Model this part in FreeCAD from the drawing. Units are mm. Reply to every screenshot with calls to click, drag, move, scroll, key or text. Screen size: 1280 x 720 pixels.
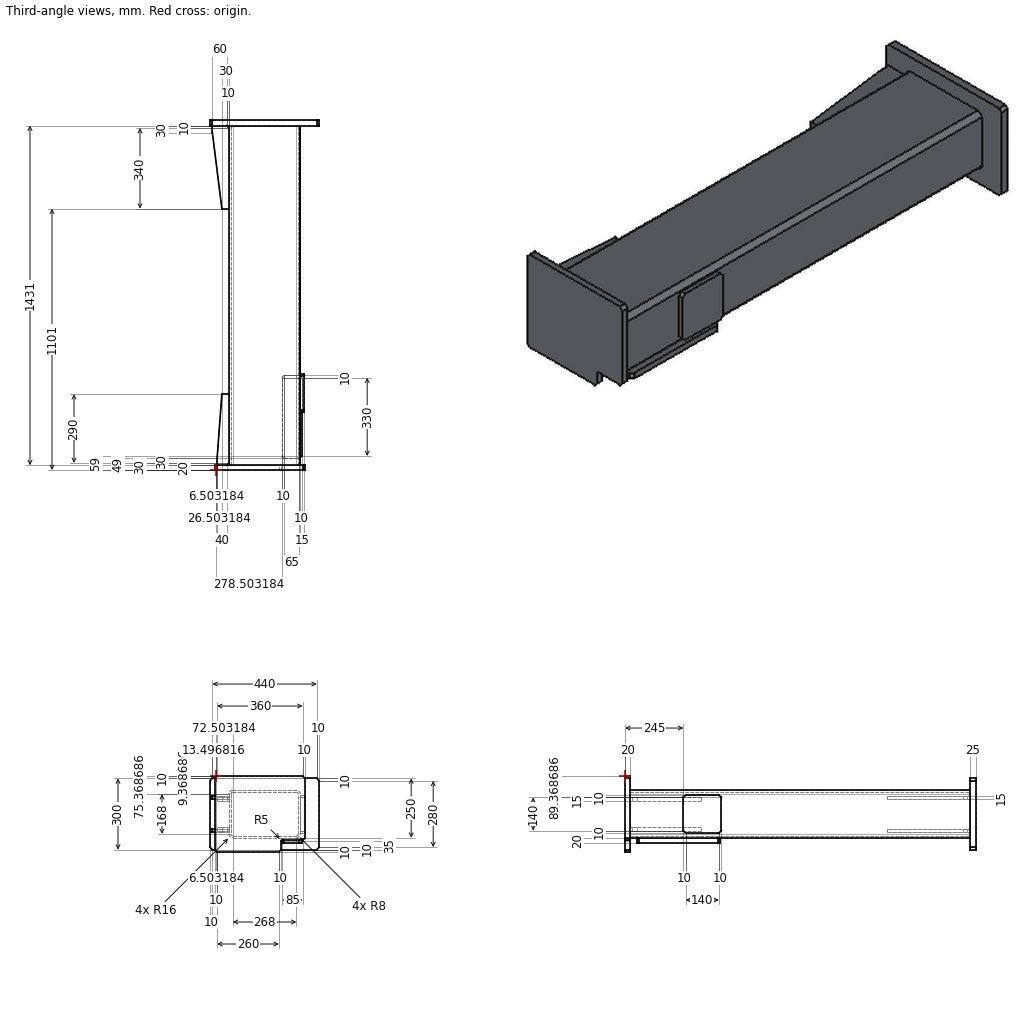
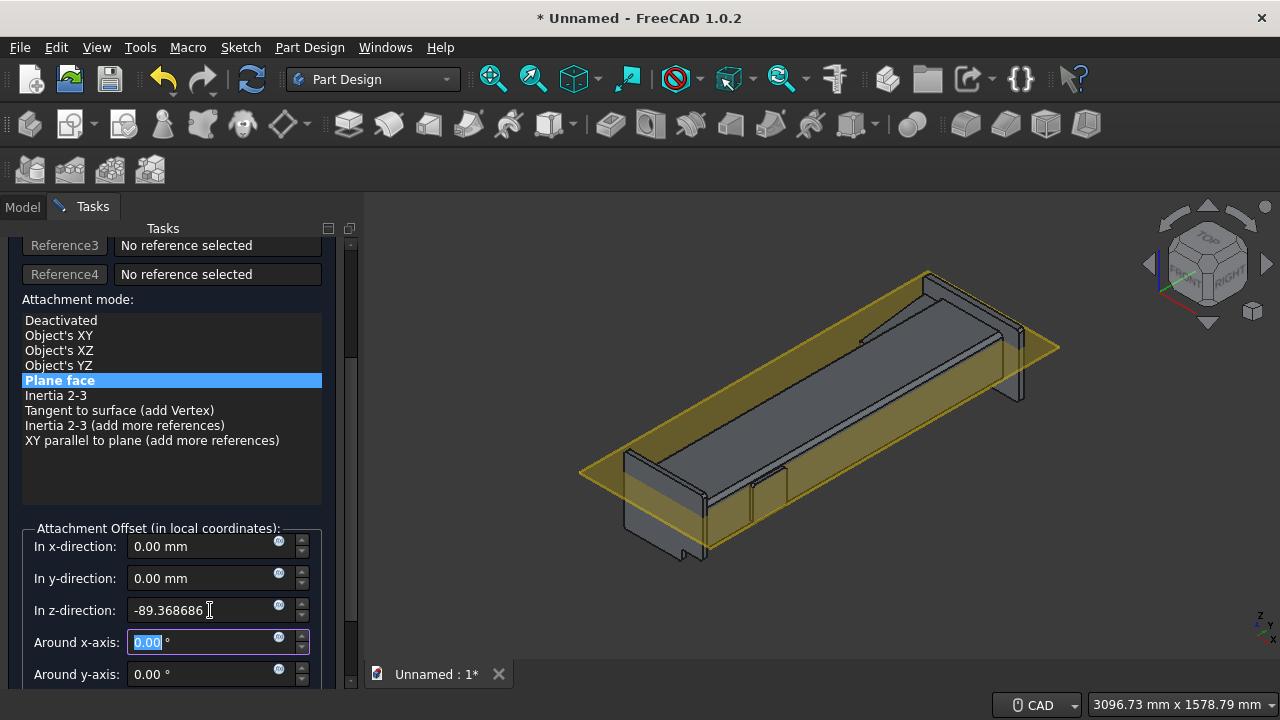
scroll(351, 463, up, 4)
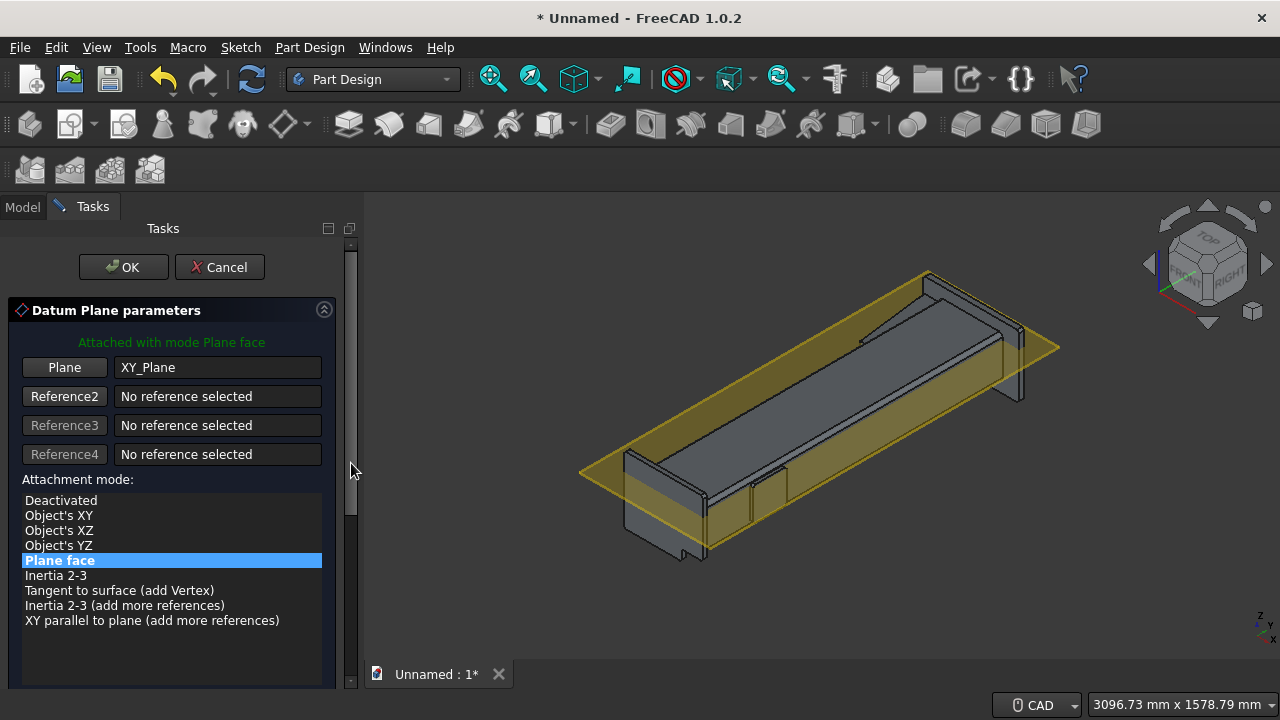
click(124, 267)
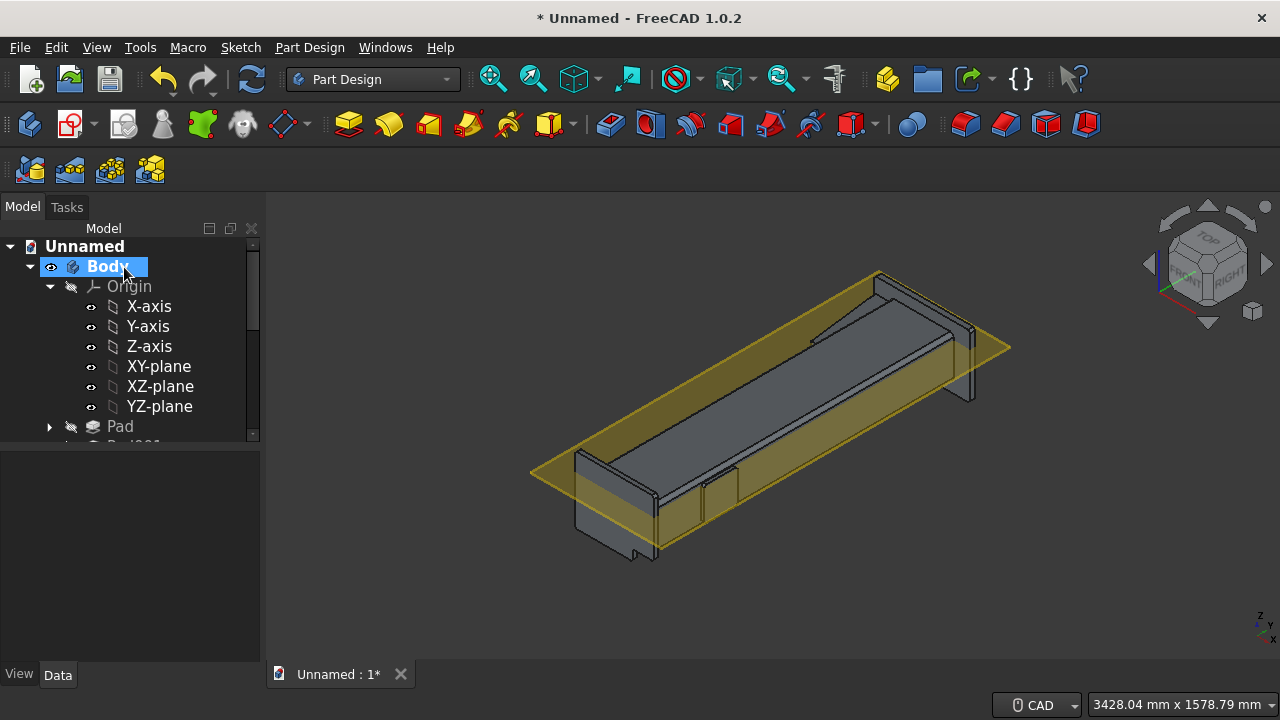
scroll(100, 342, down, 3)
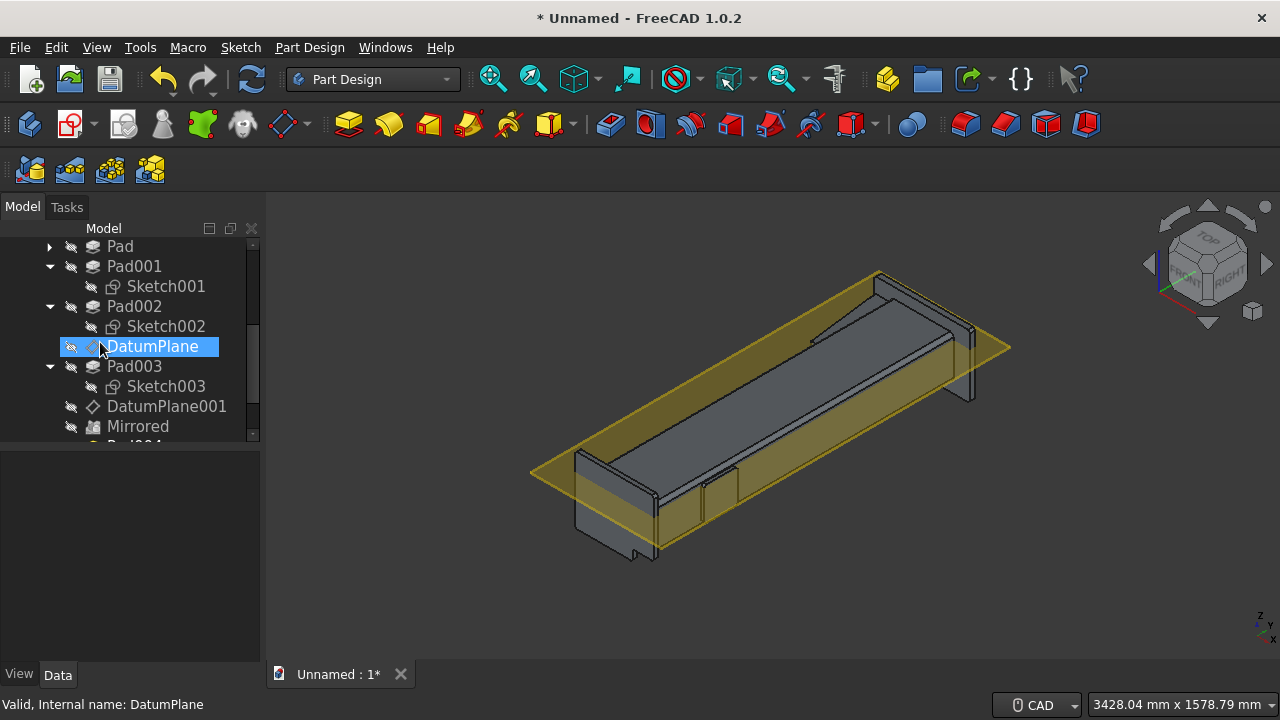
scroll(140, 342, up, 15)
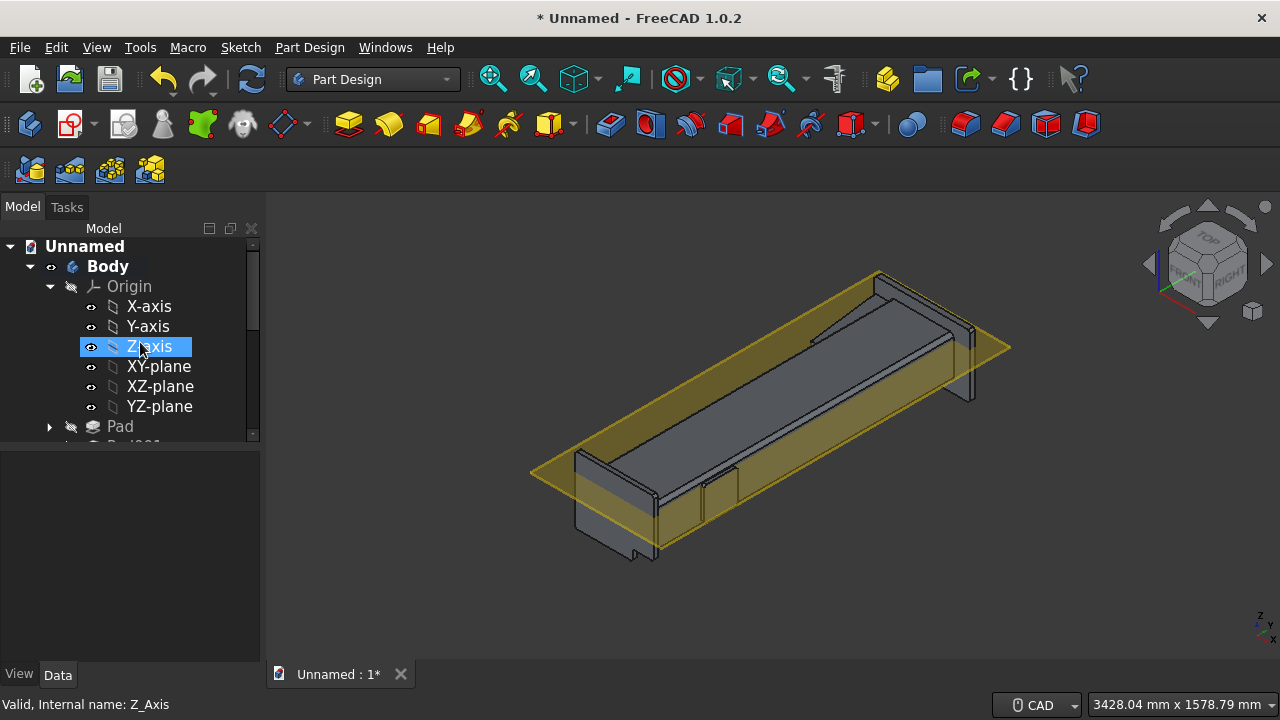
scroll(100, 342, down, 6)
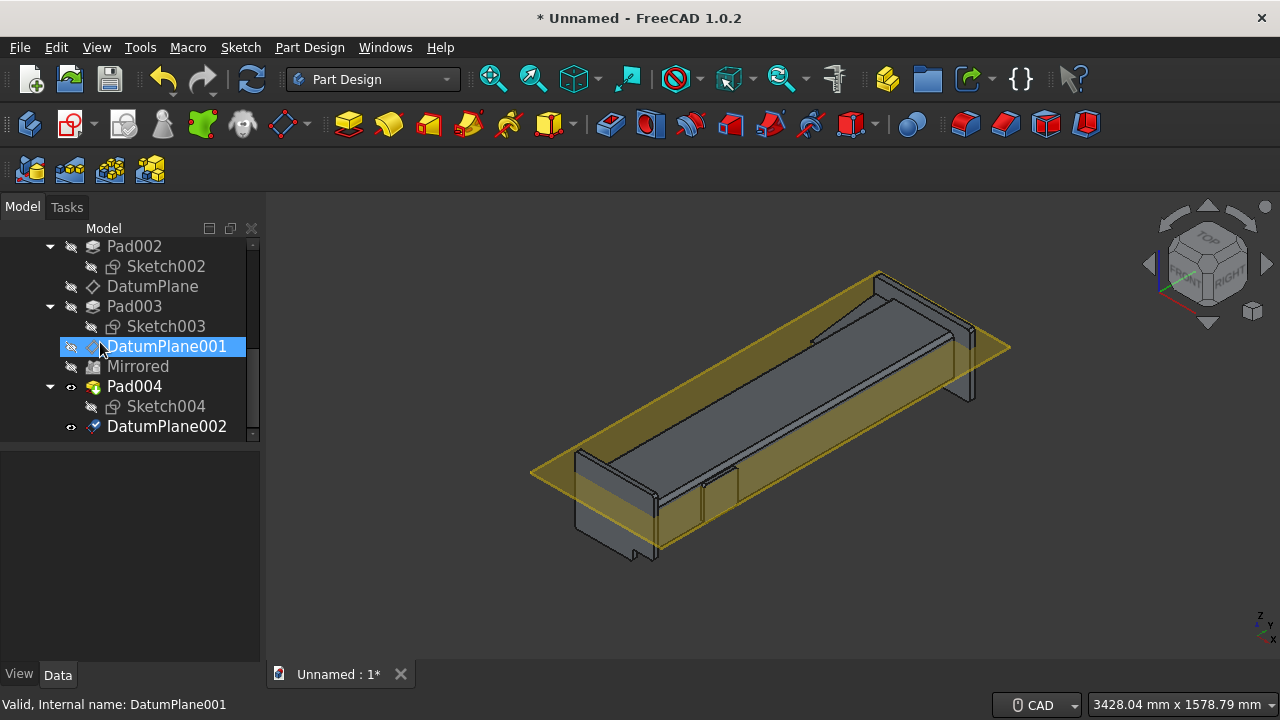
click(116, 427)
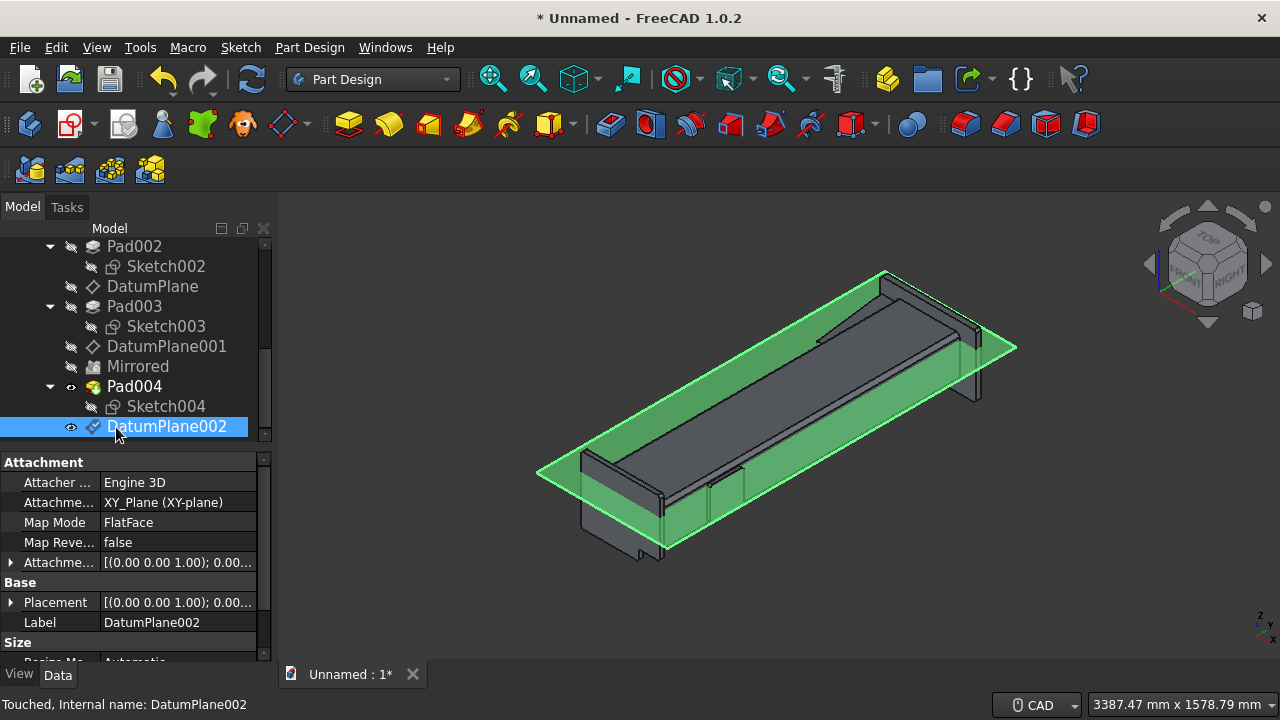
click(70, 124)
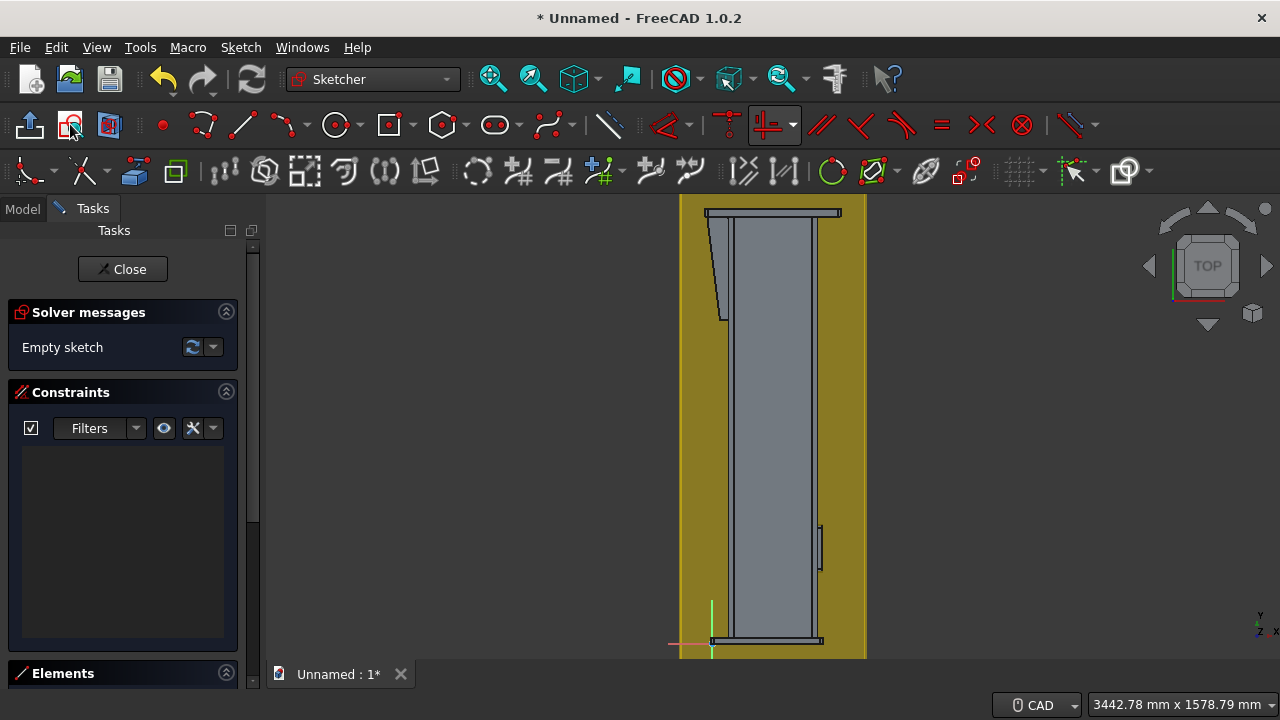
click(110, 126)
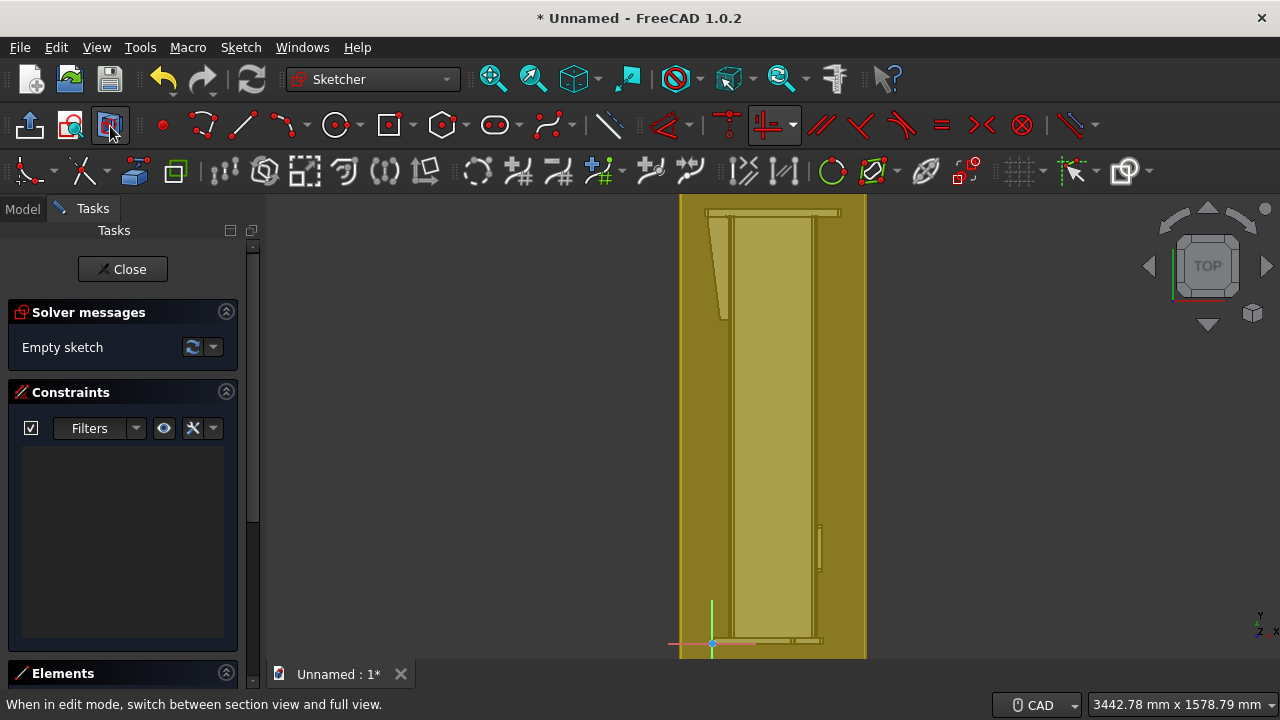
scroll(704, 426, down, 5)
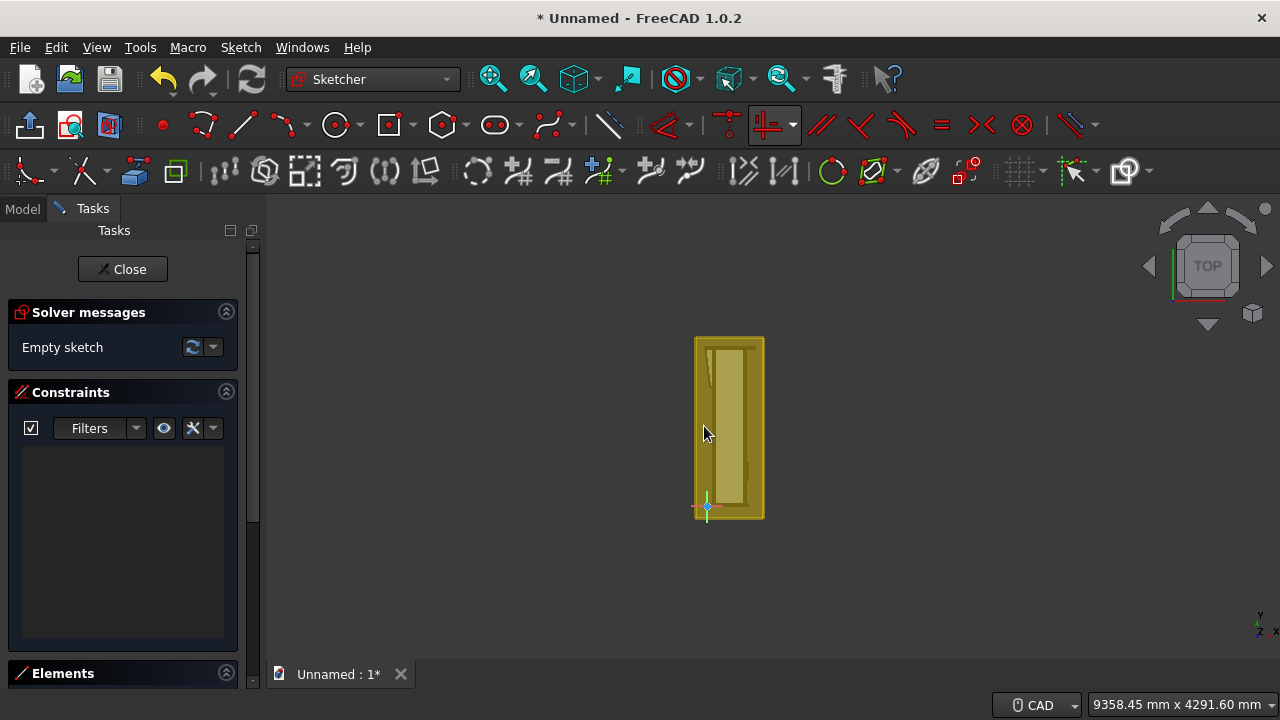
scroll(711, 497, up, 11)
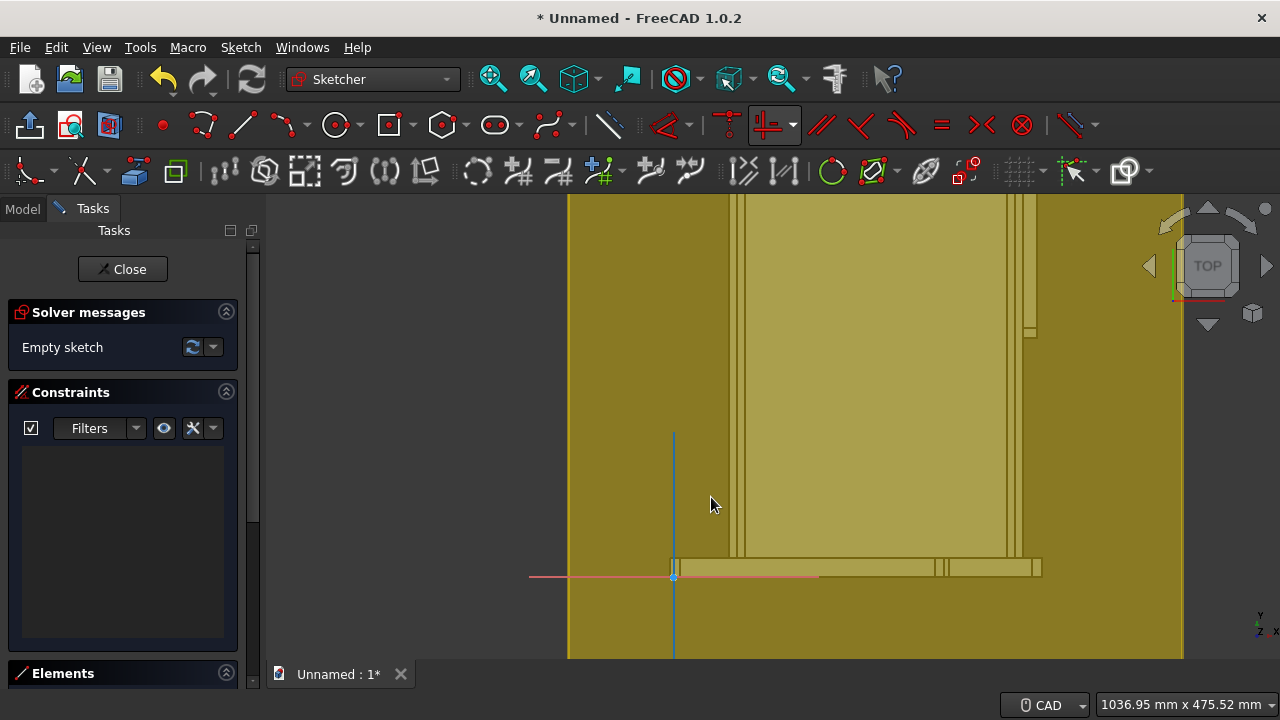
key(g)
key(m)